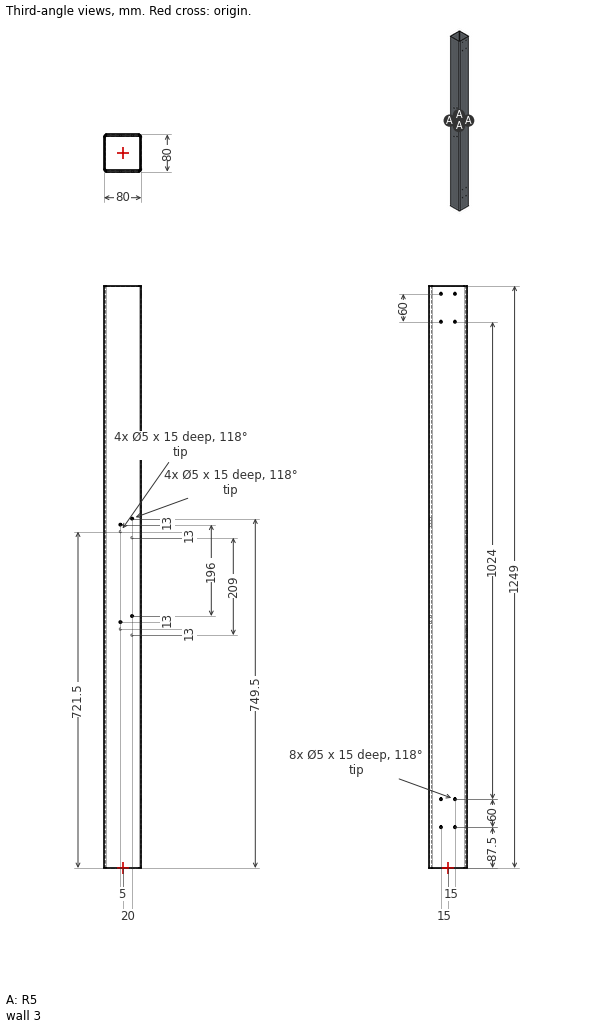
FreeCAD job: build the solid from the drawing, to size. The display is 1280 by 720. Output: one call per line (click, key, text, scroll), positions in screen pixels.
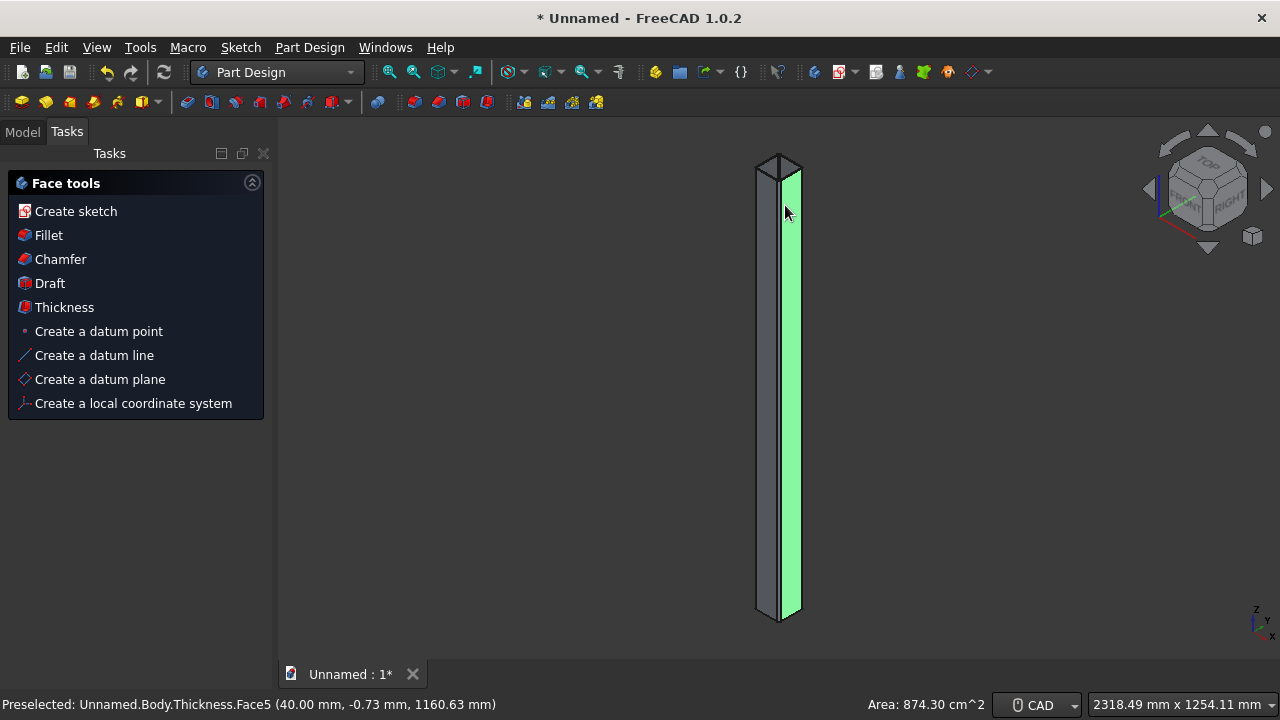
click(840, 72)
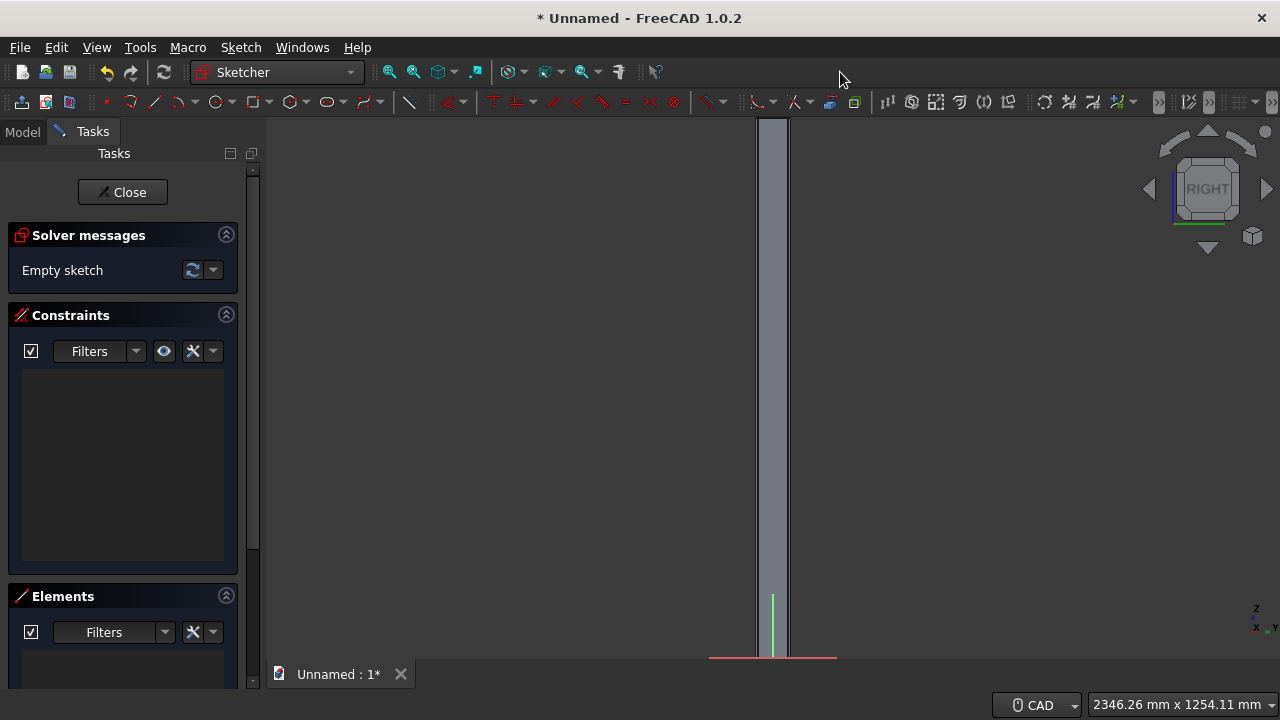
scroll(565, 381, down, 2)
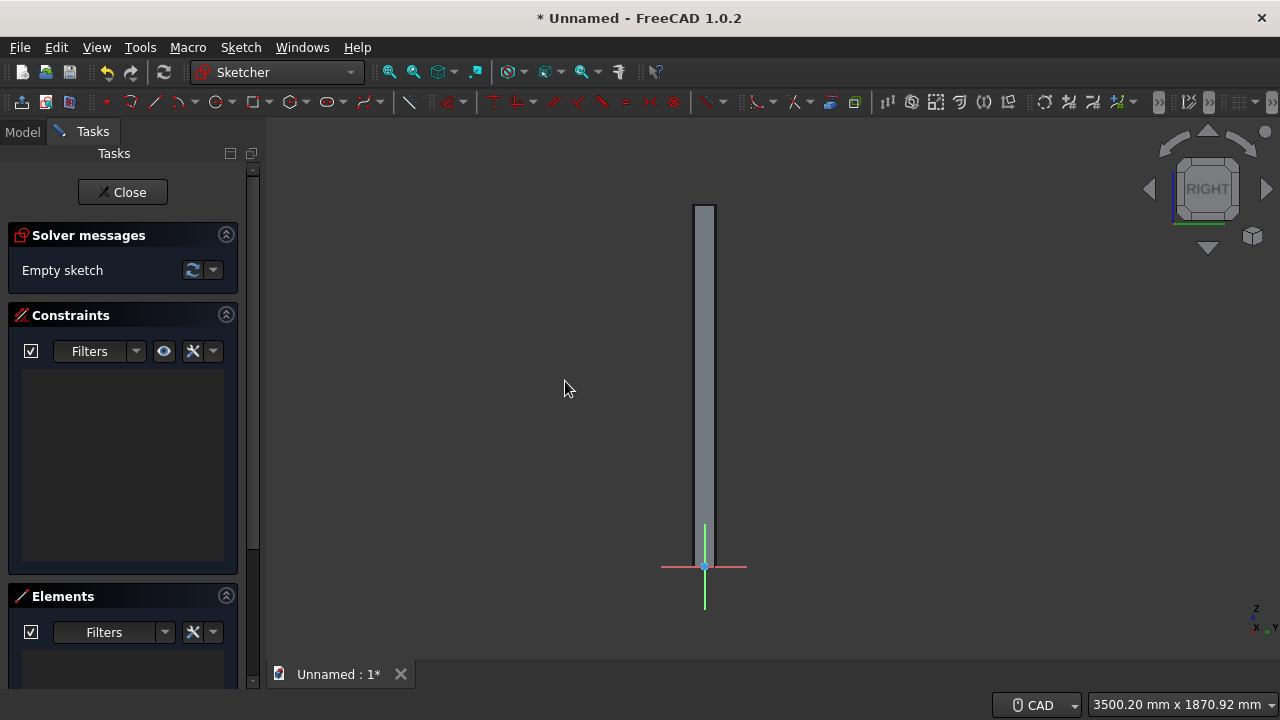
key(g)
key(c)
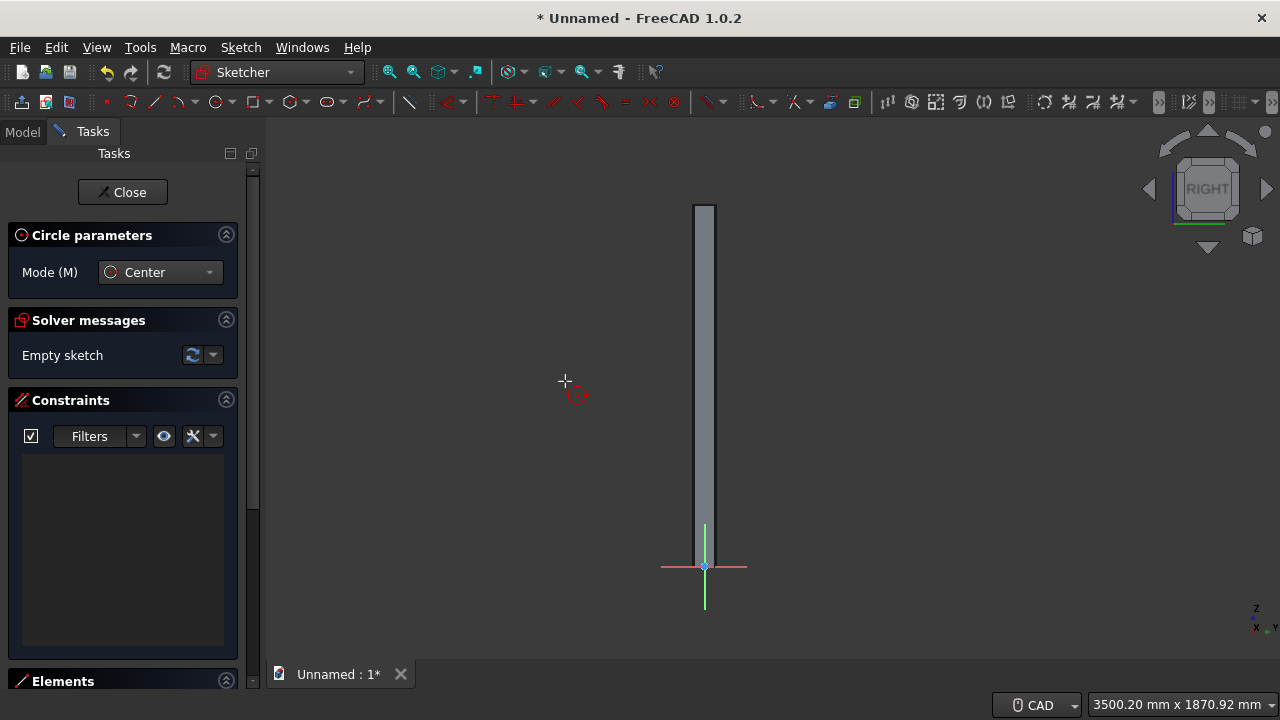
scroll(709, 524, up, 18)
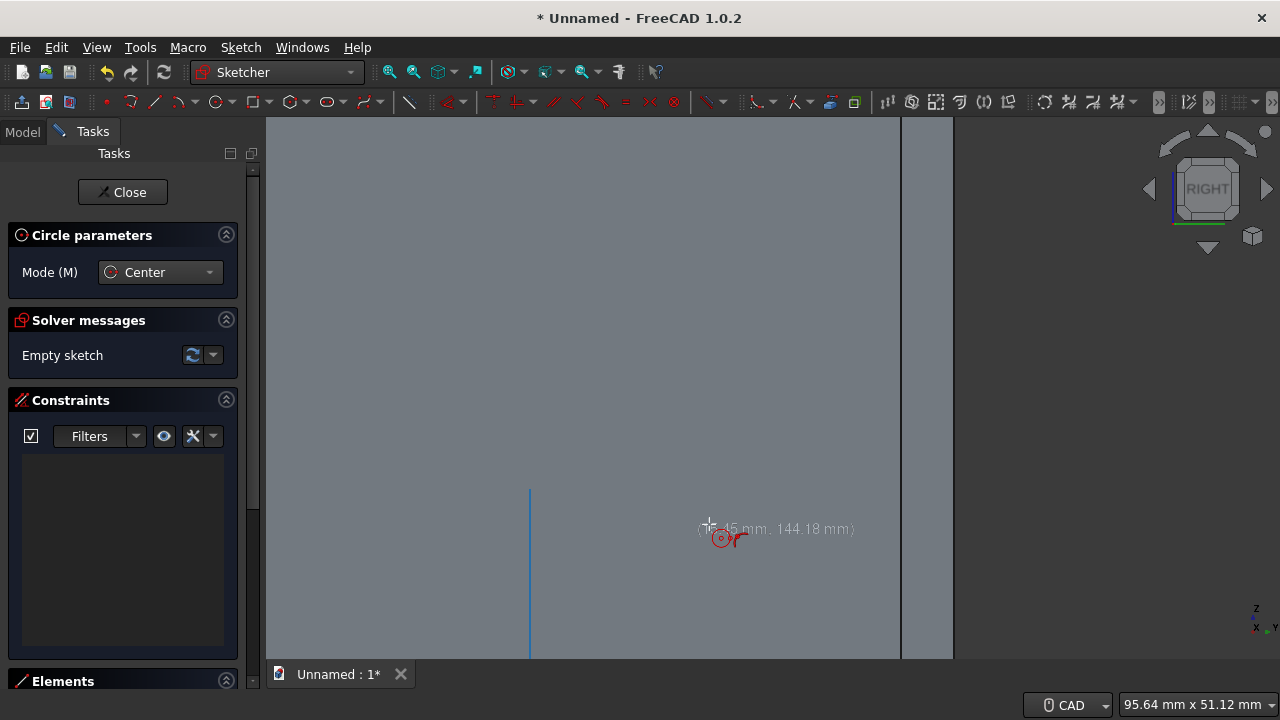
scroll(709, 525, down, 18)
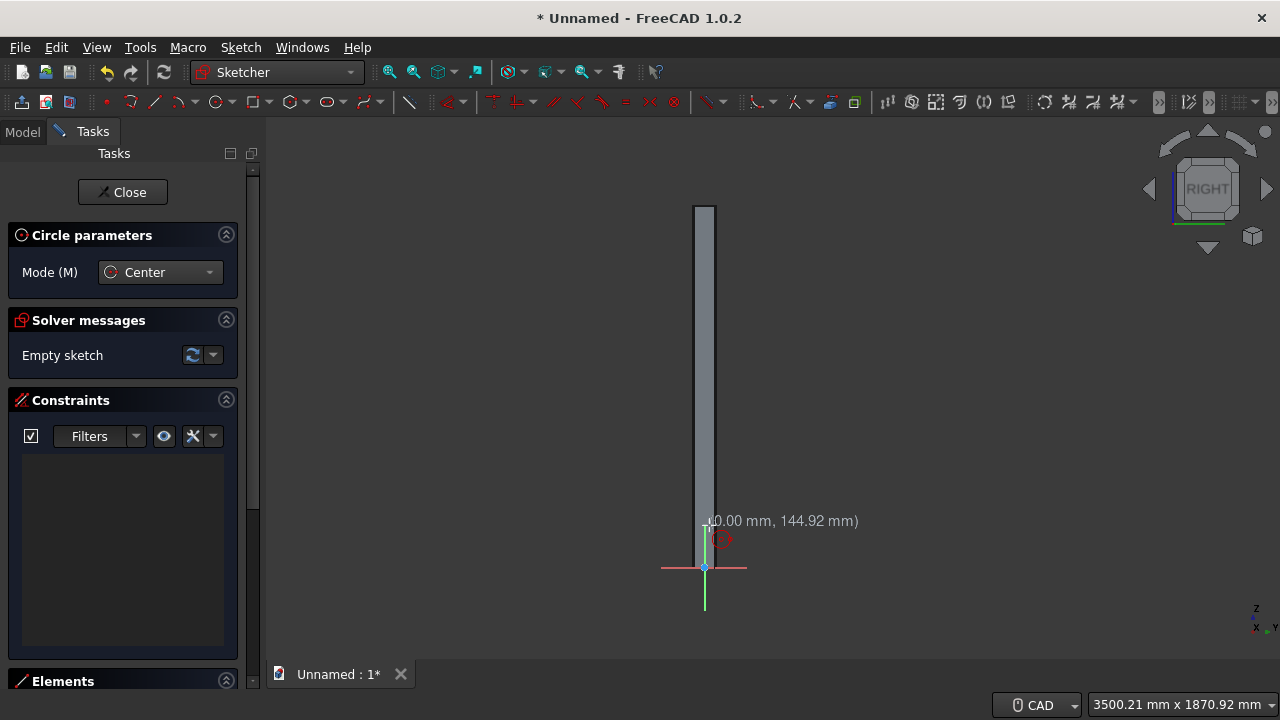
scroll(709, 525, up, 7)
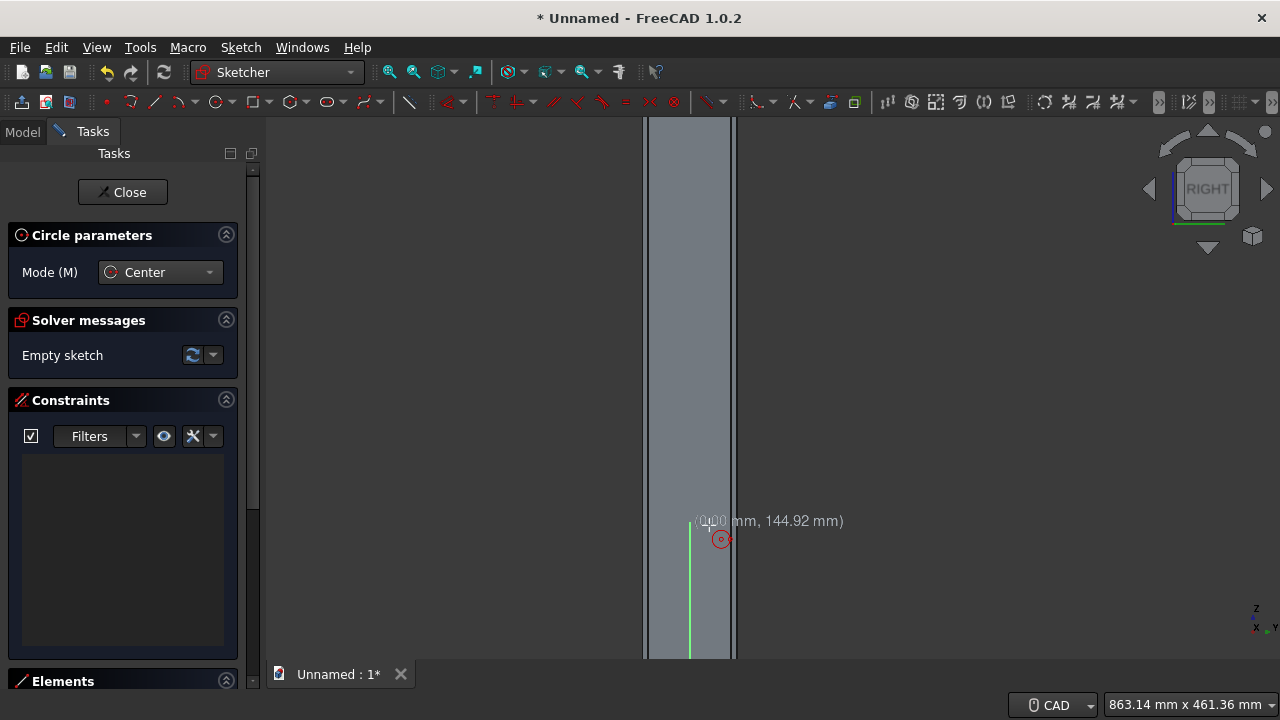
click(707, 523)
move(709, 521)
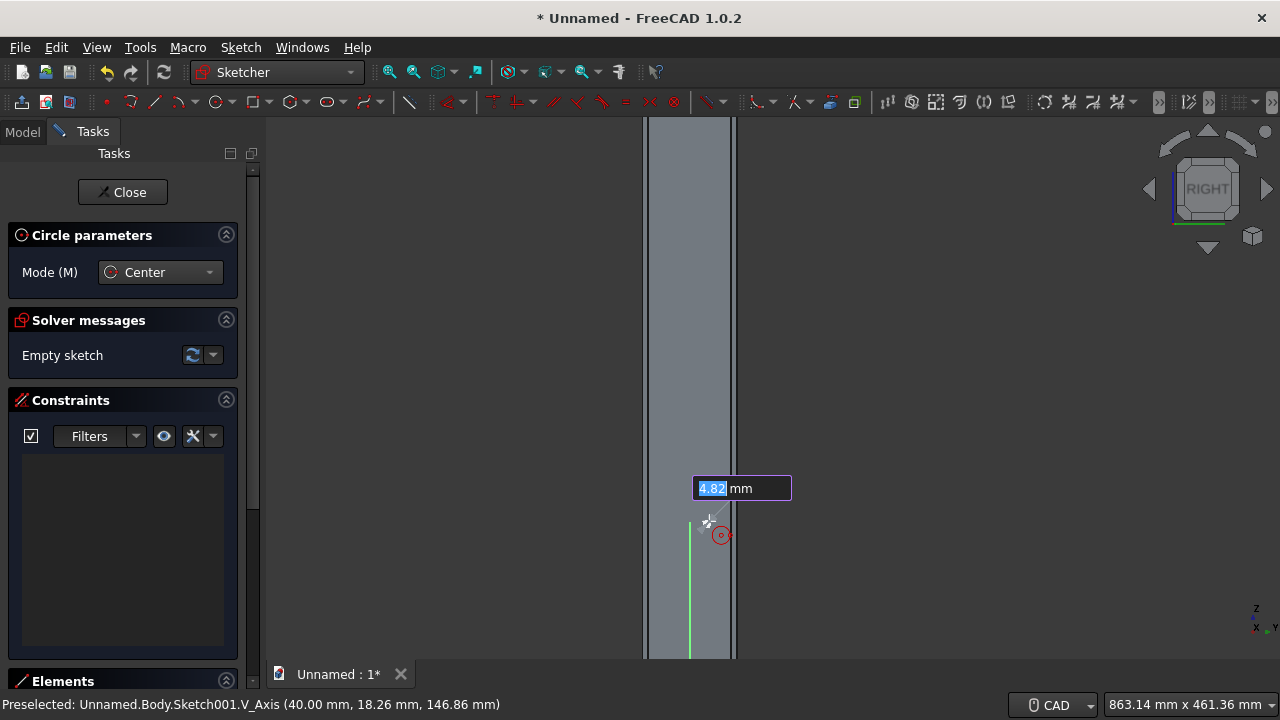
text(5)
key(Return)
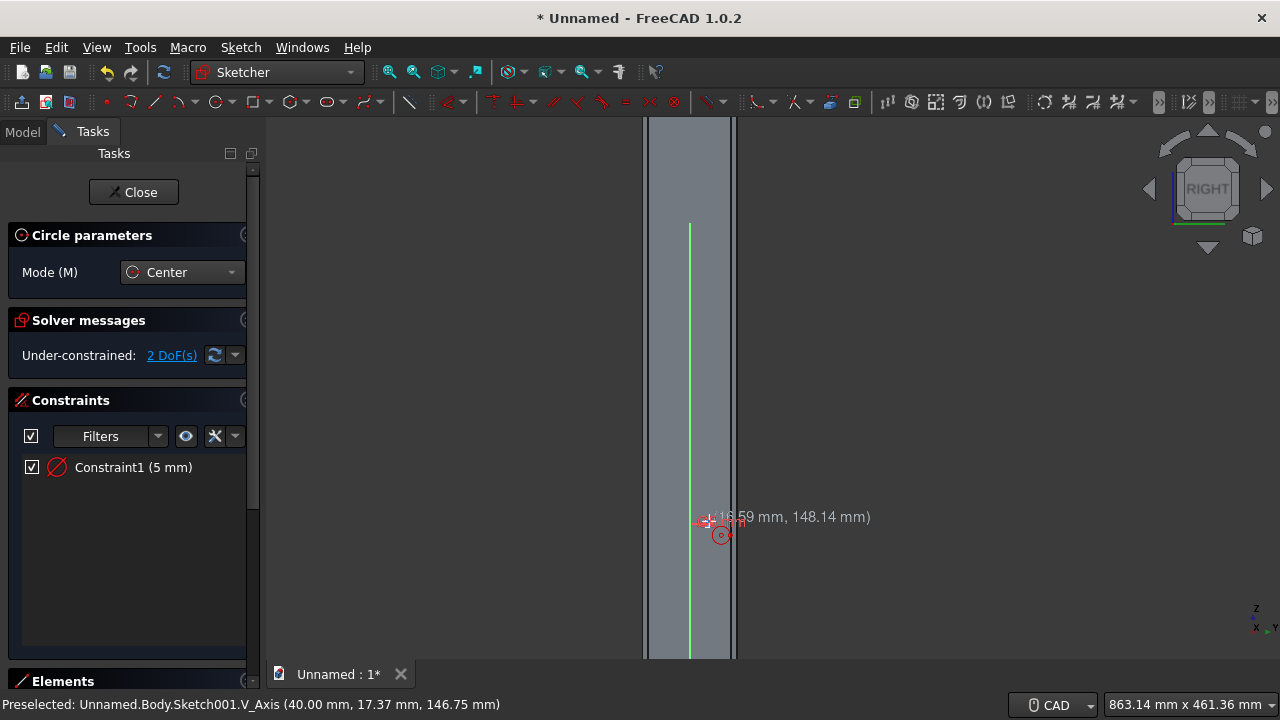
scroll(707, 593, up, 11)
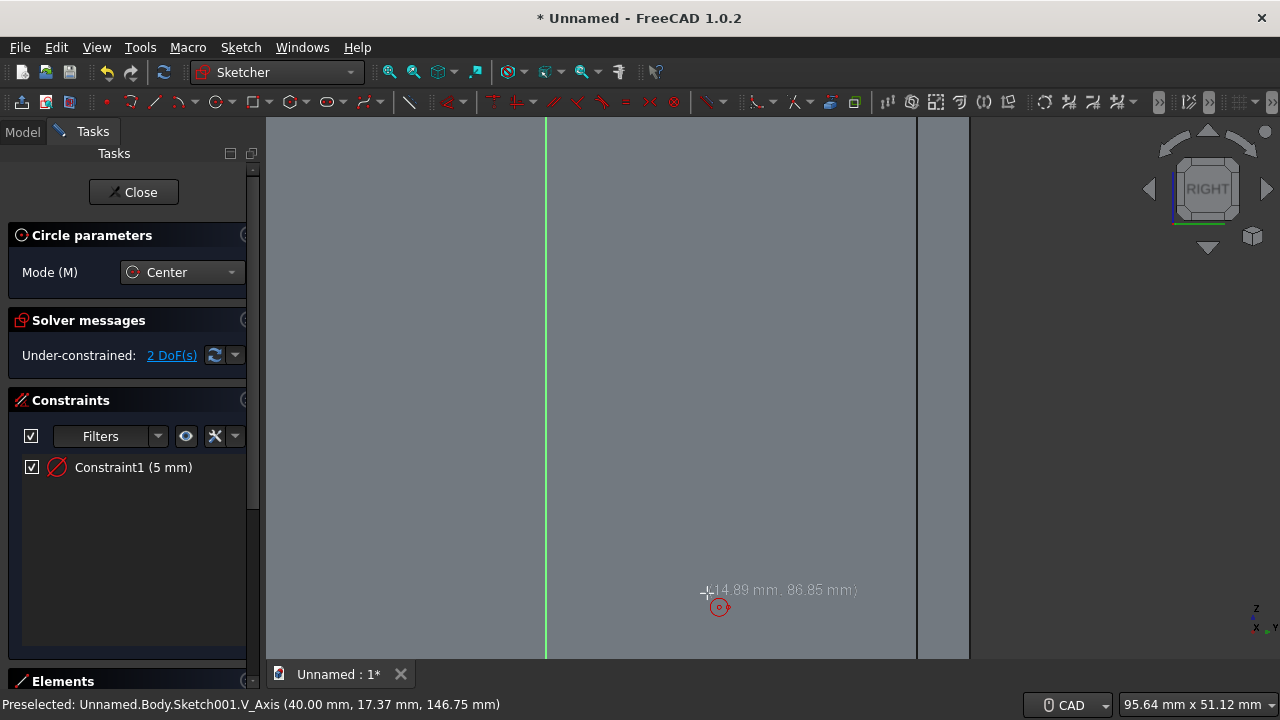
scroll(709, 540, down, 18)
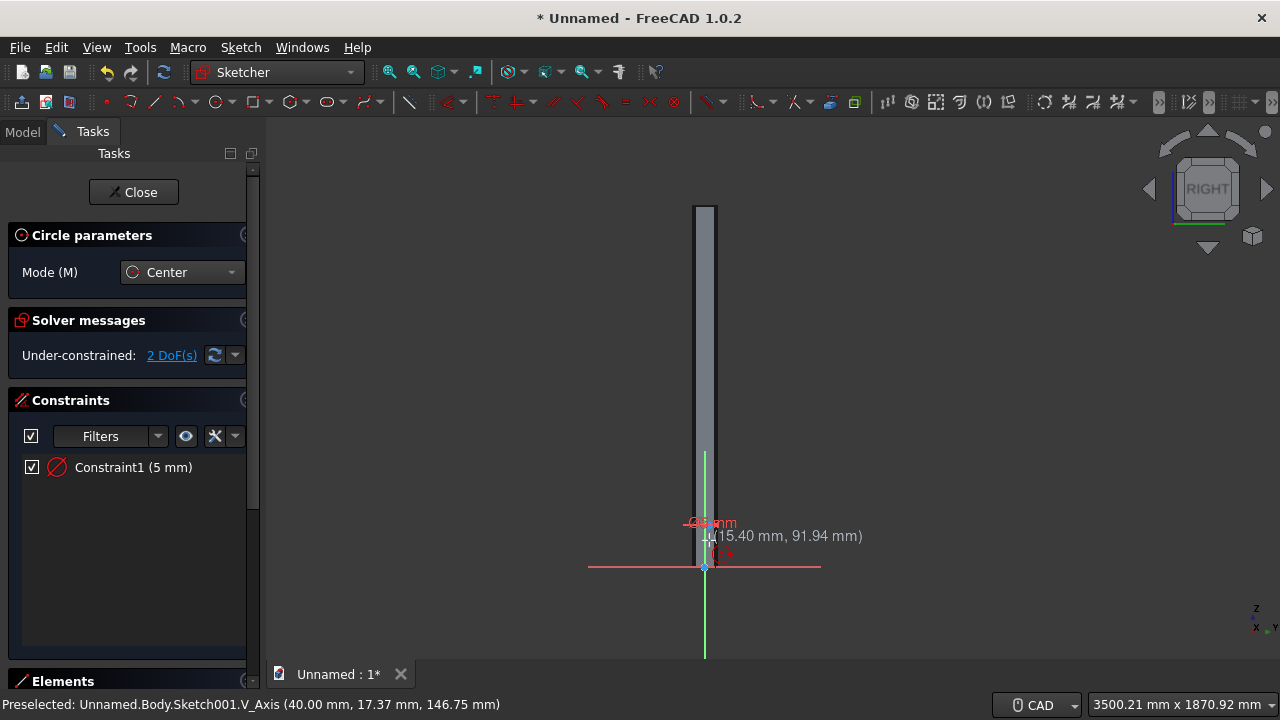
scroll(709, 542, up, 7)